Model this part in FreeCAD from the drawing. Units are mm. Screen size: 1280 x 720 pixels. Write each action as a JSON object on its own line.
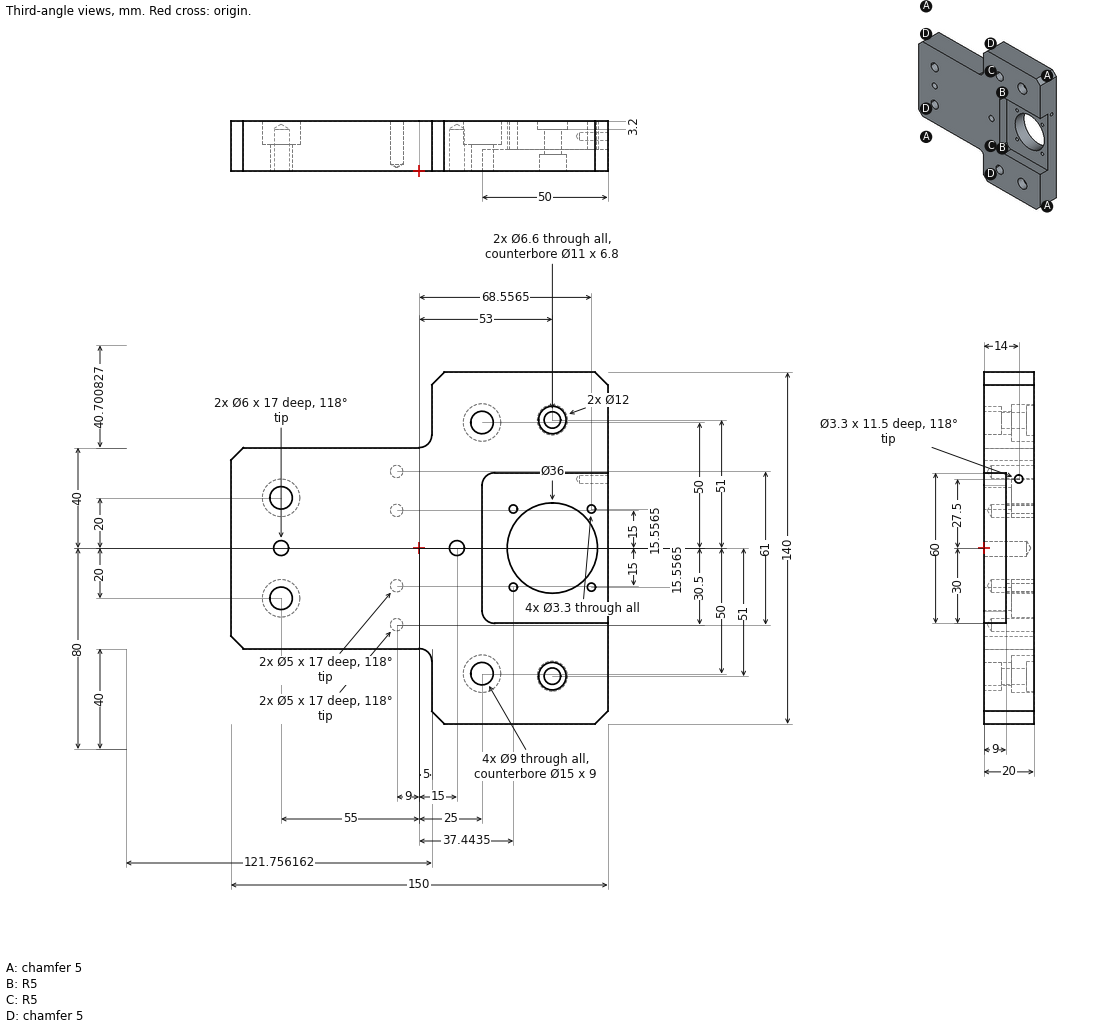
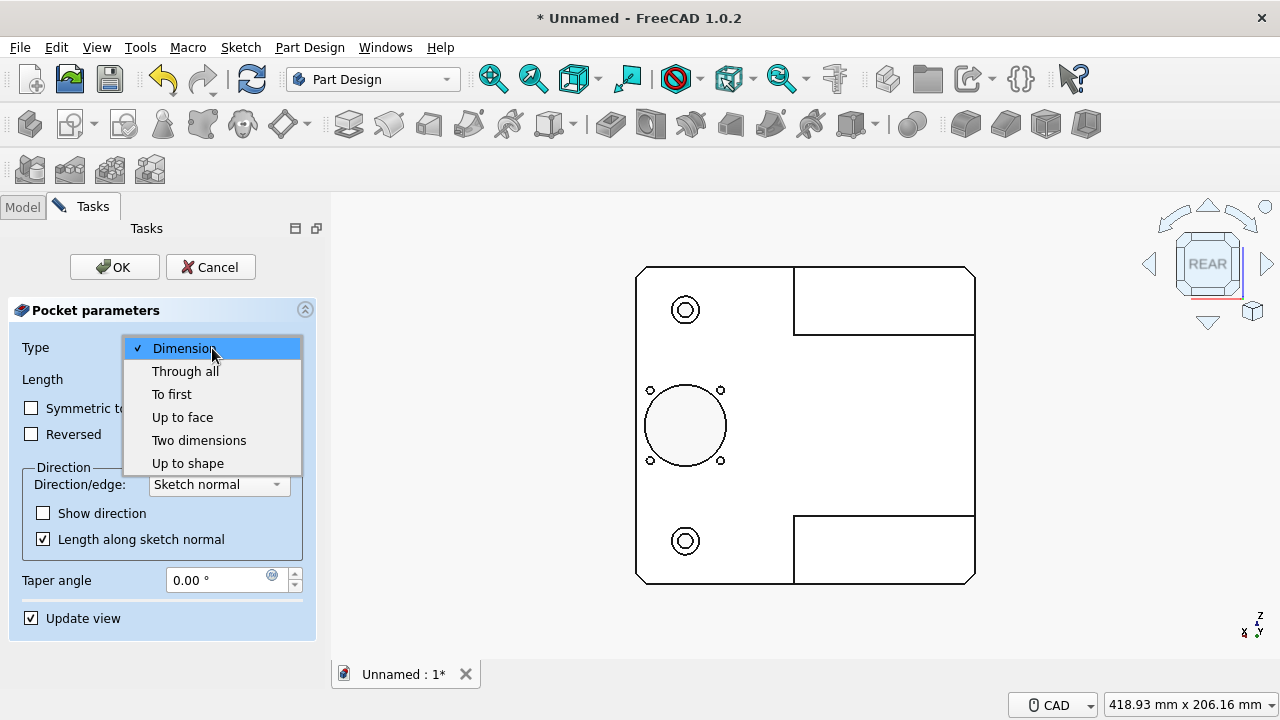
{"action": "left_click", "coordinate": [212, 372]}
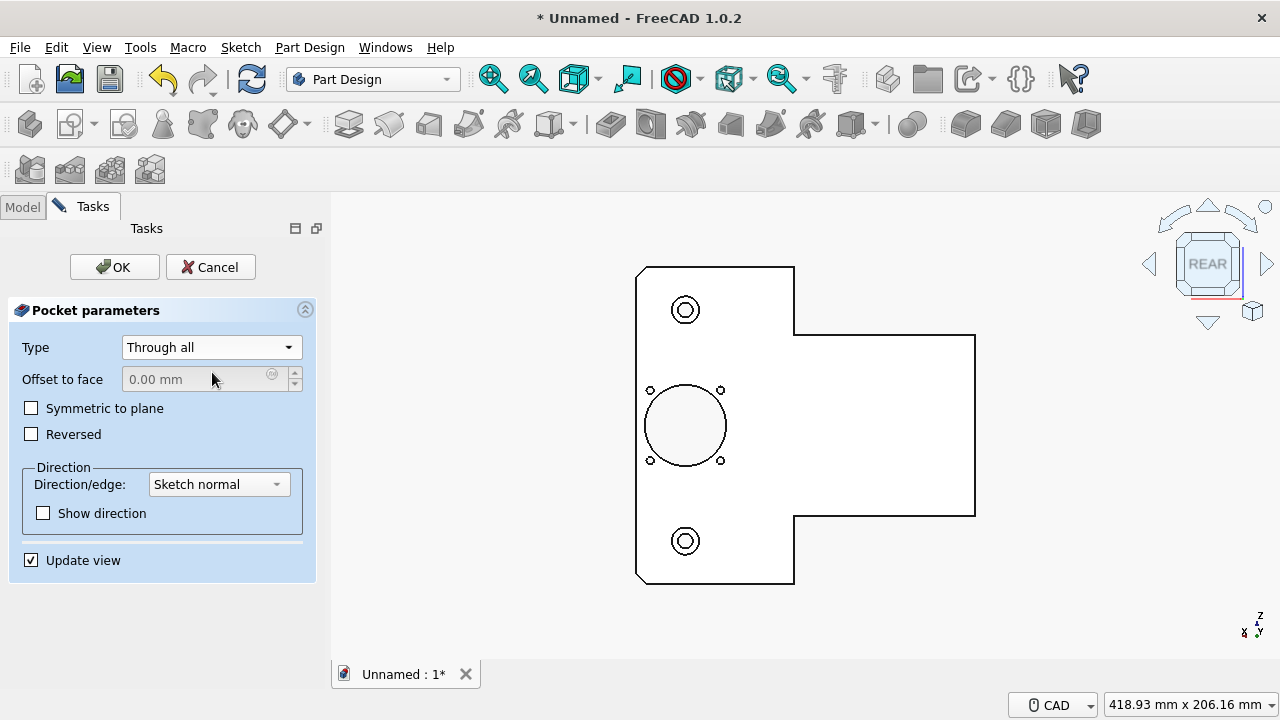
{"action": "left_click", "coordinate": [115, 267]}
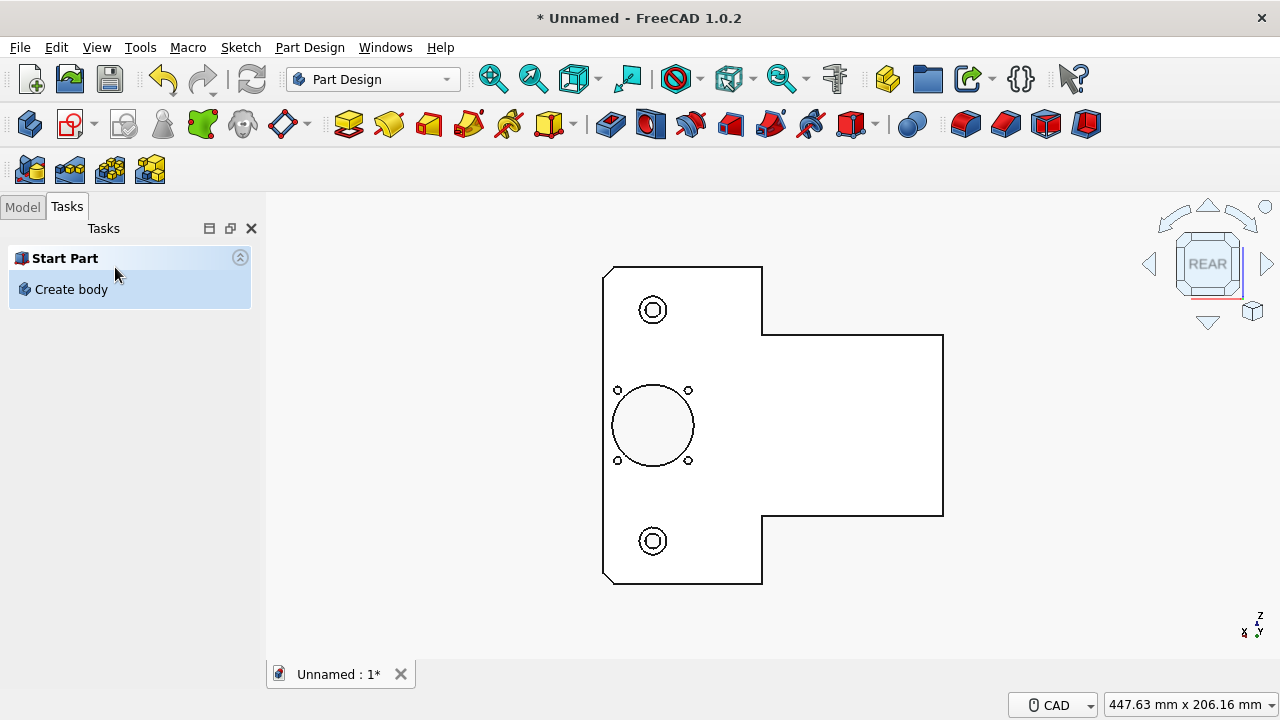
{"action": "key", "text": "0"}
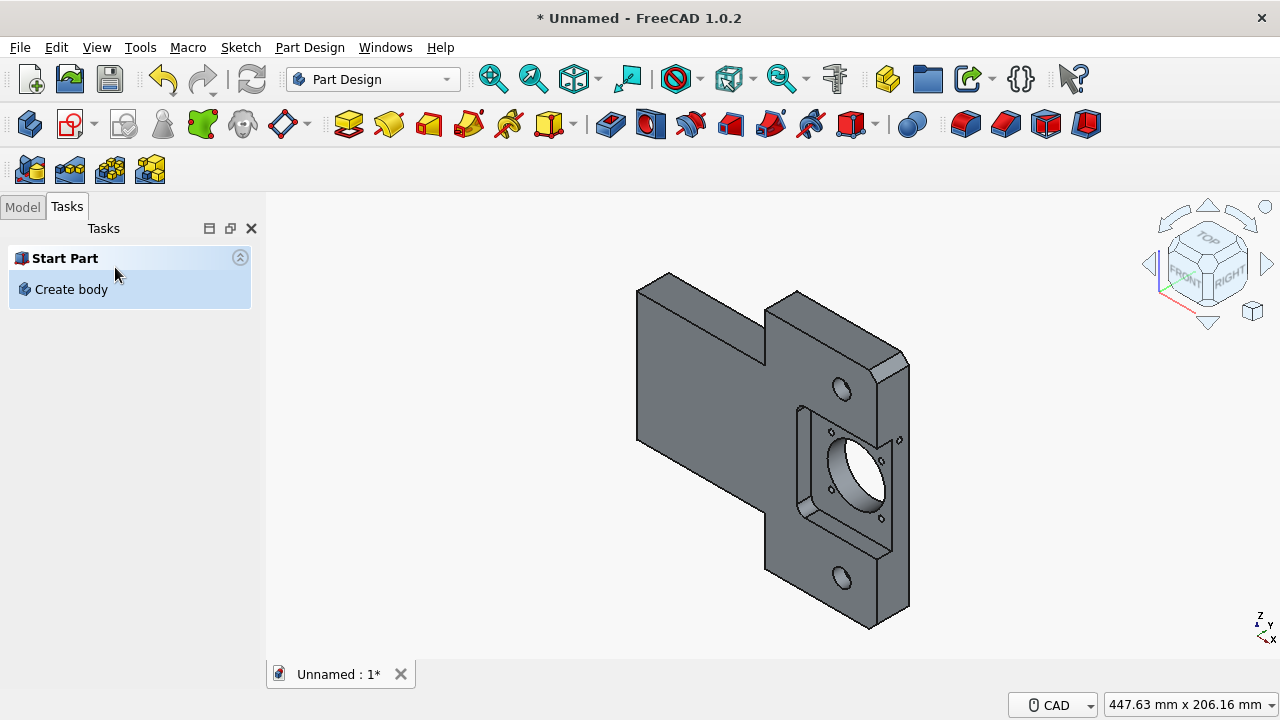
{"action": "key", "text": "2"}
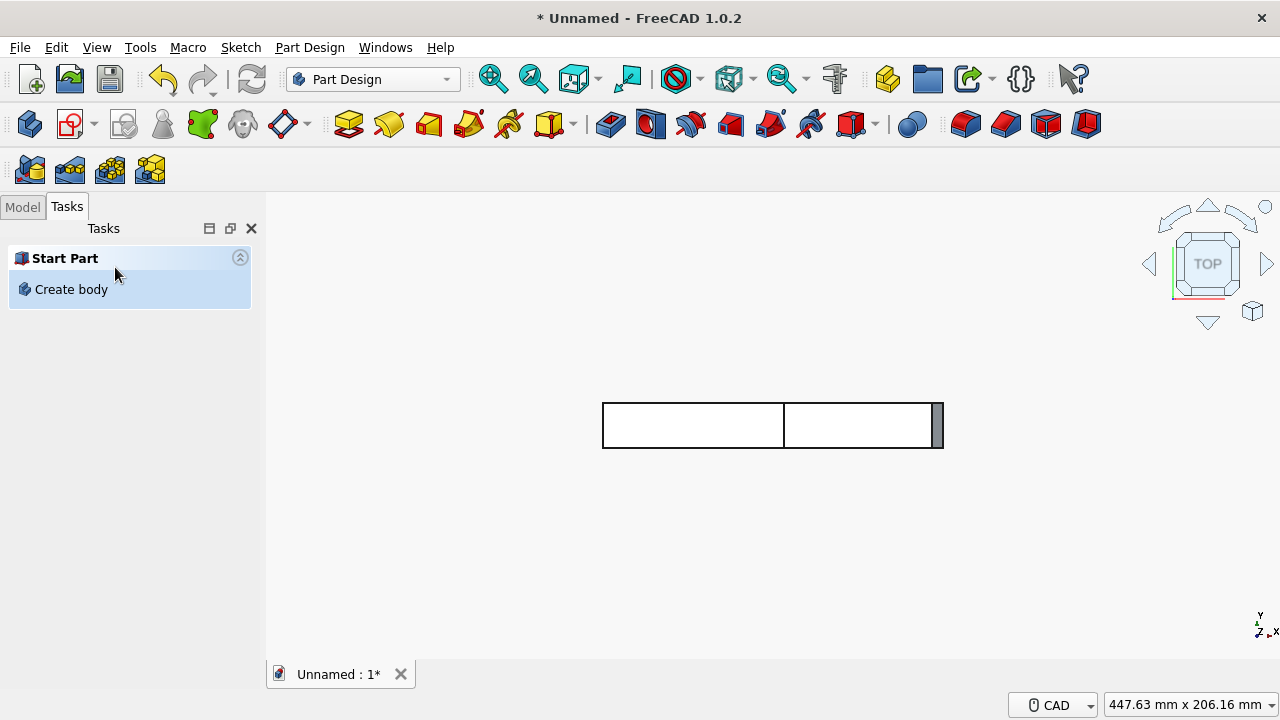
{"action": "left_click", "coordinate": [494, 80]}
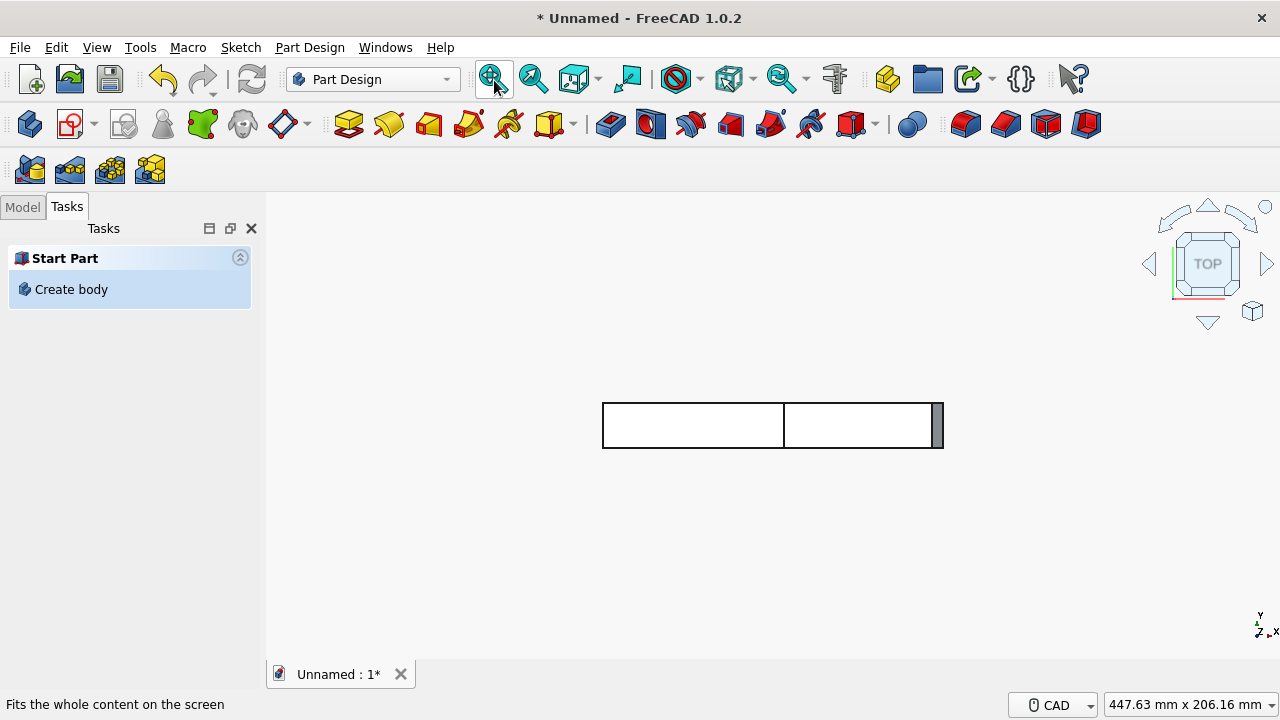
{"action": "key", "text": "1"}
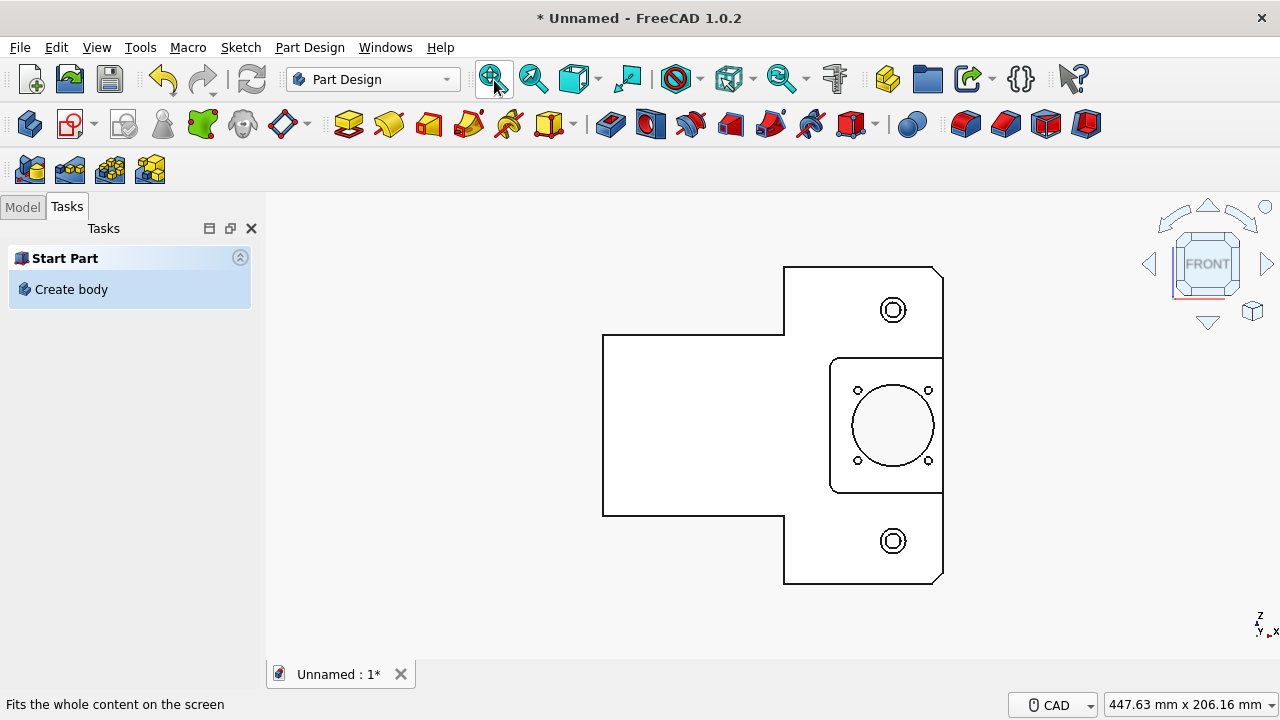
{"action": "key", "text": "3"}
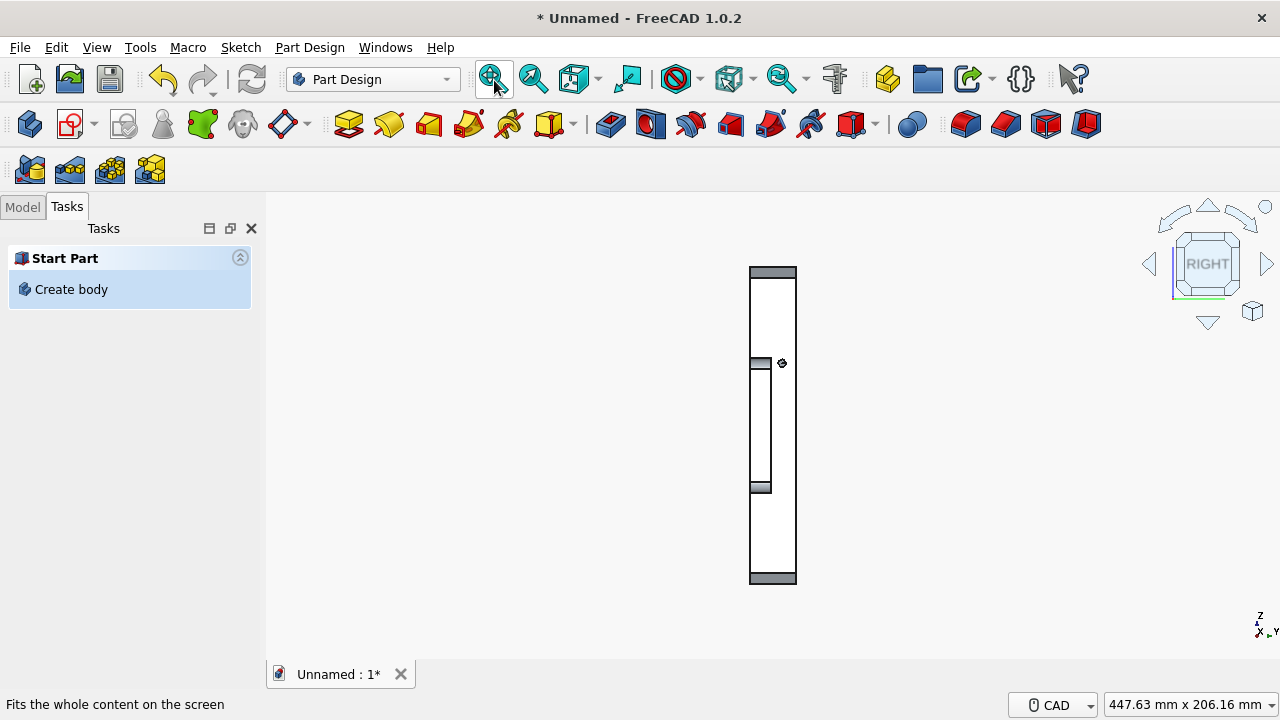
{"action": "key", "text": "5"}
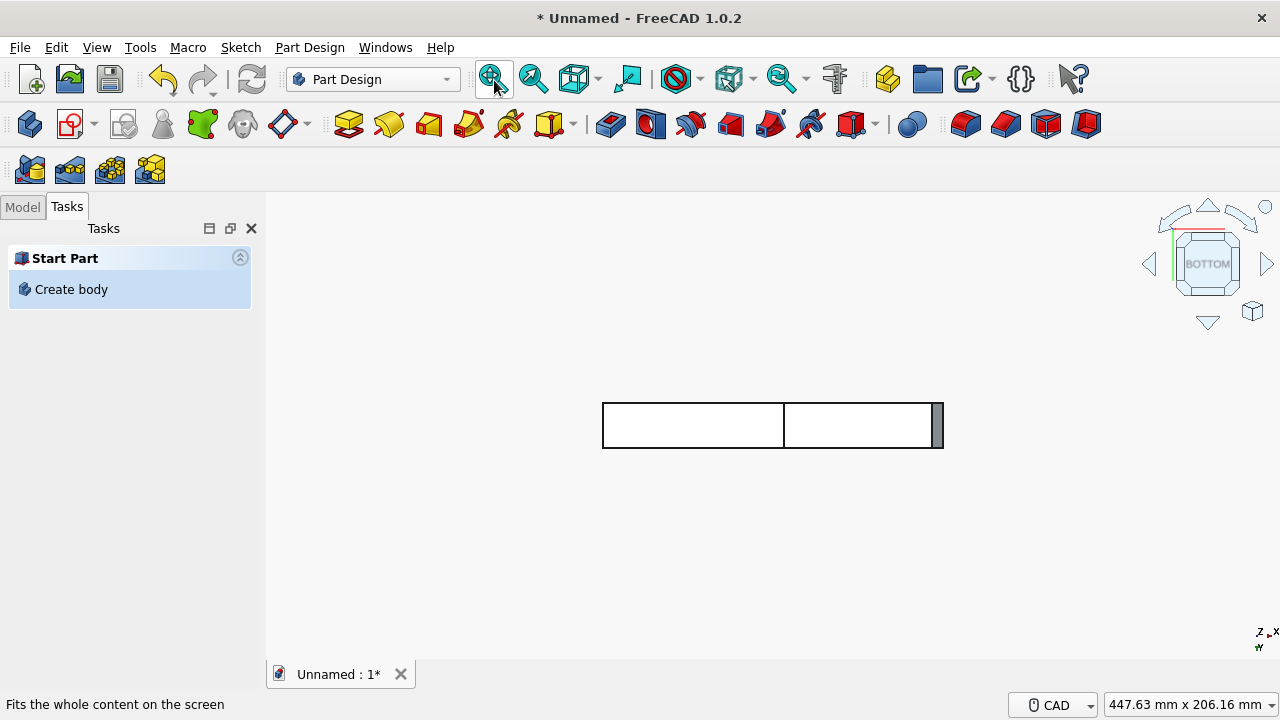
{"action": "left_click", "coordinate": [494, 80]}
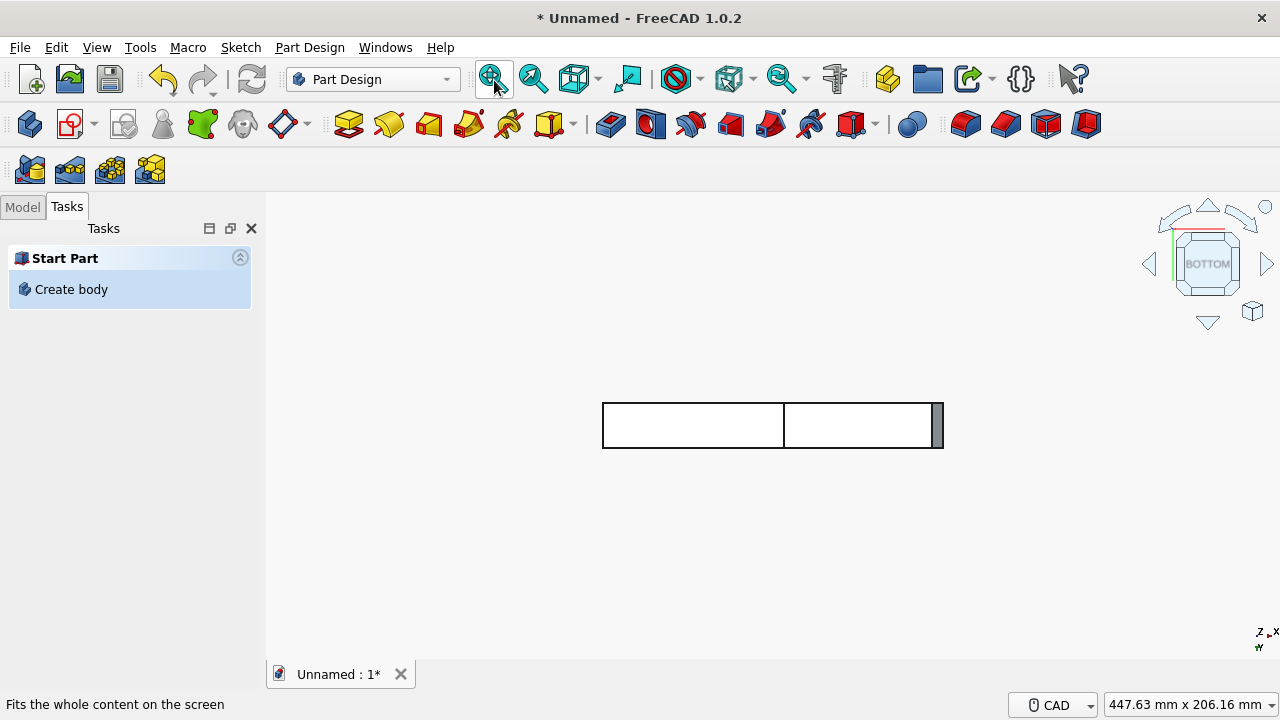
{"action": "key", "text": "4"}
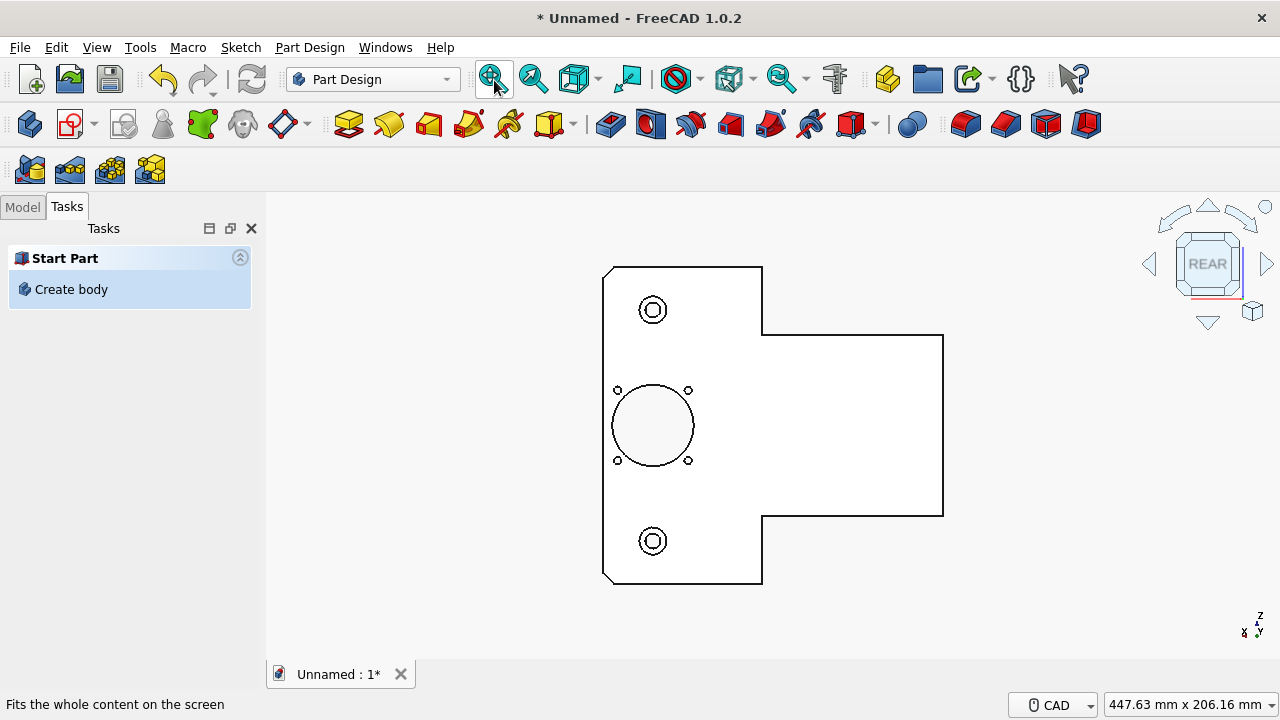
{"action": "key", "text": "6"}